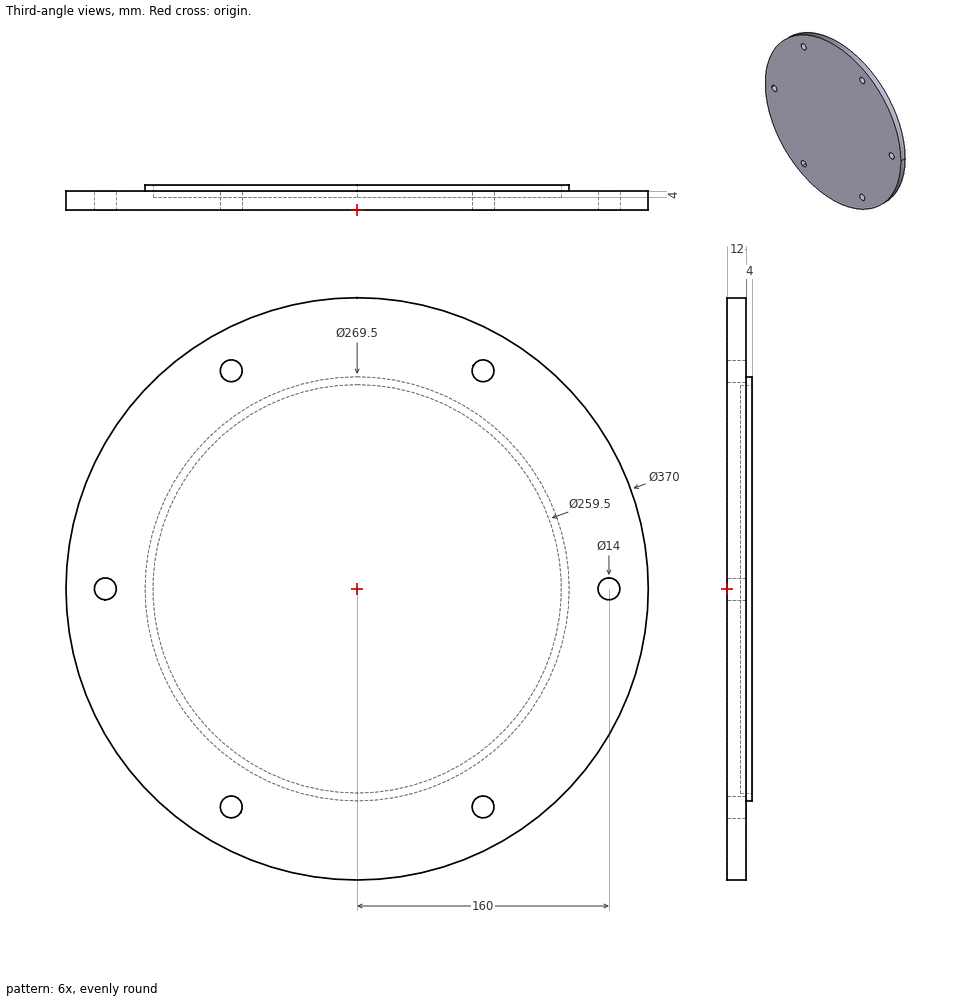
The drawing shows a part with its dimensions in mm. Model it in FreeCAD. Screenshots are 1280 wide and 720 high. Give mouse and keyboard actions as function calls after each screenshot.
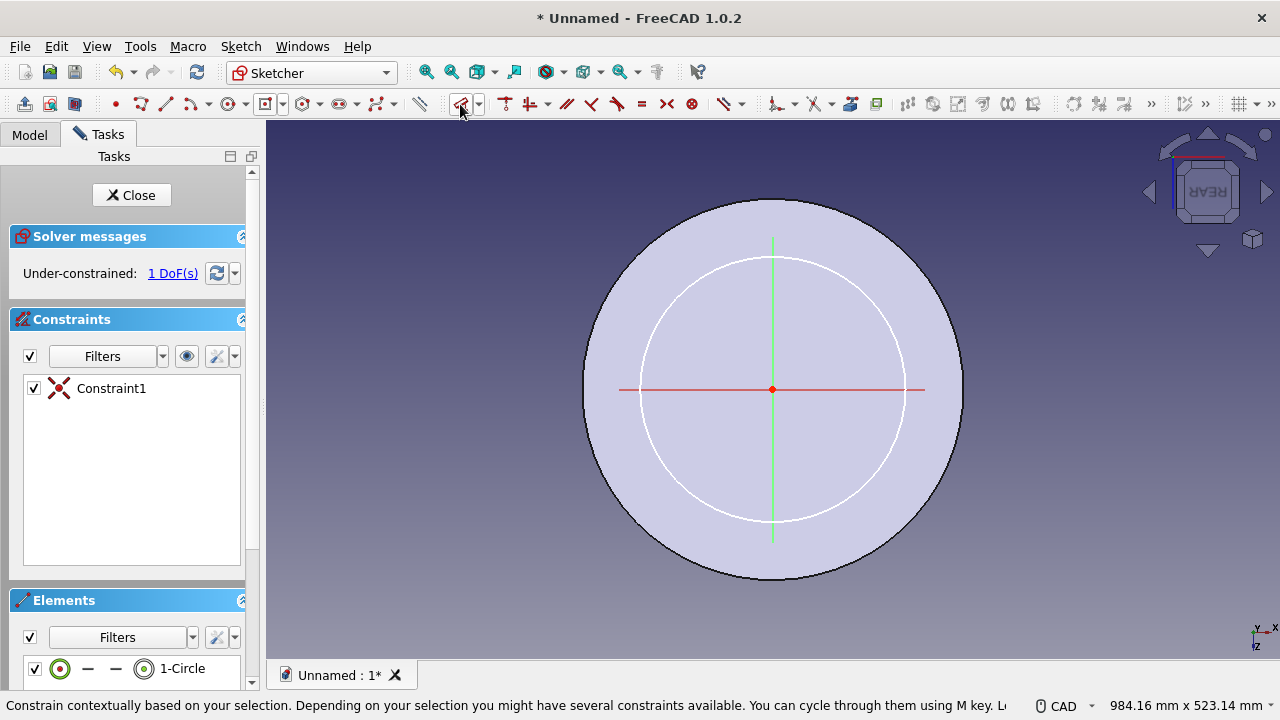
click(866, 295)
click(888, 272)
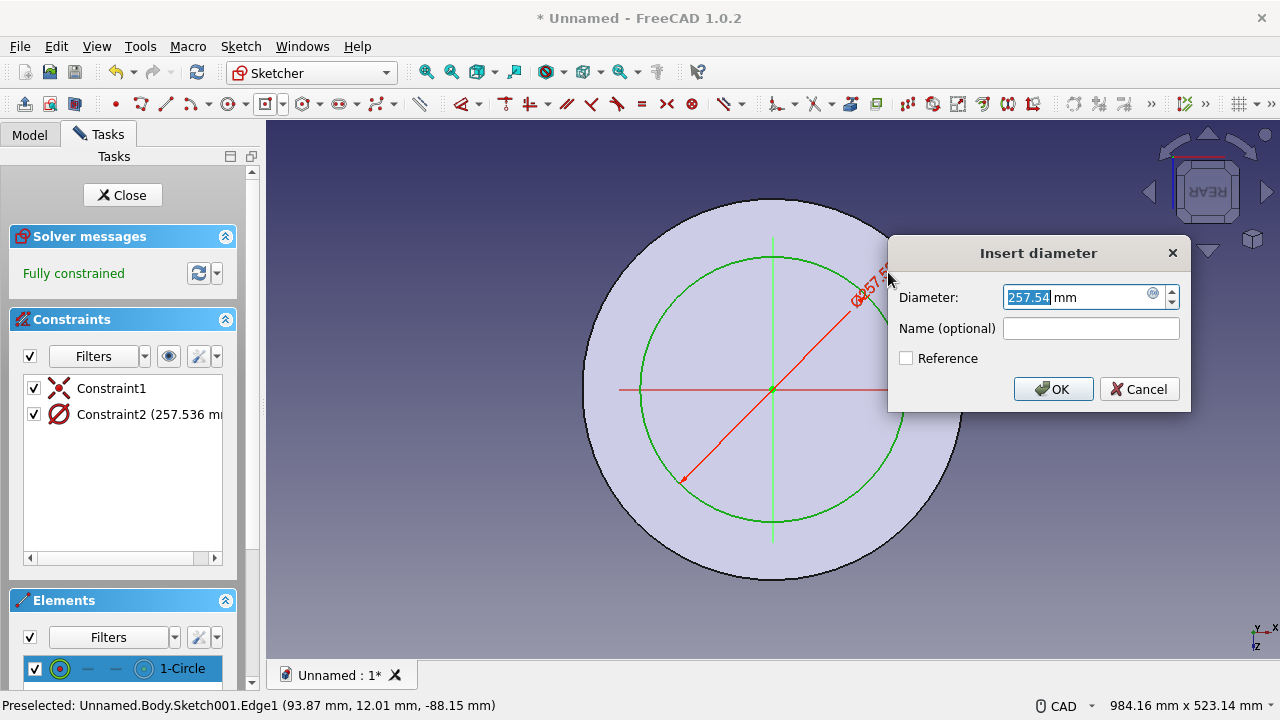
text(259.5)
key(Return)
key(Escape)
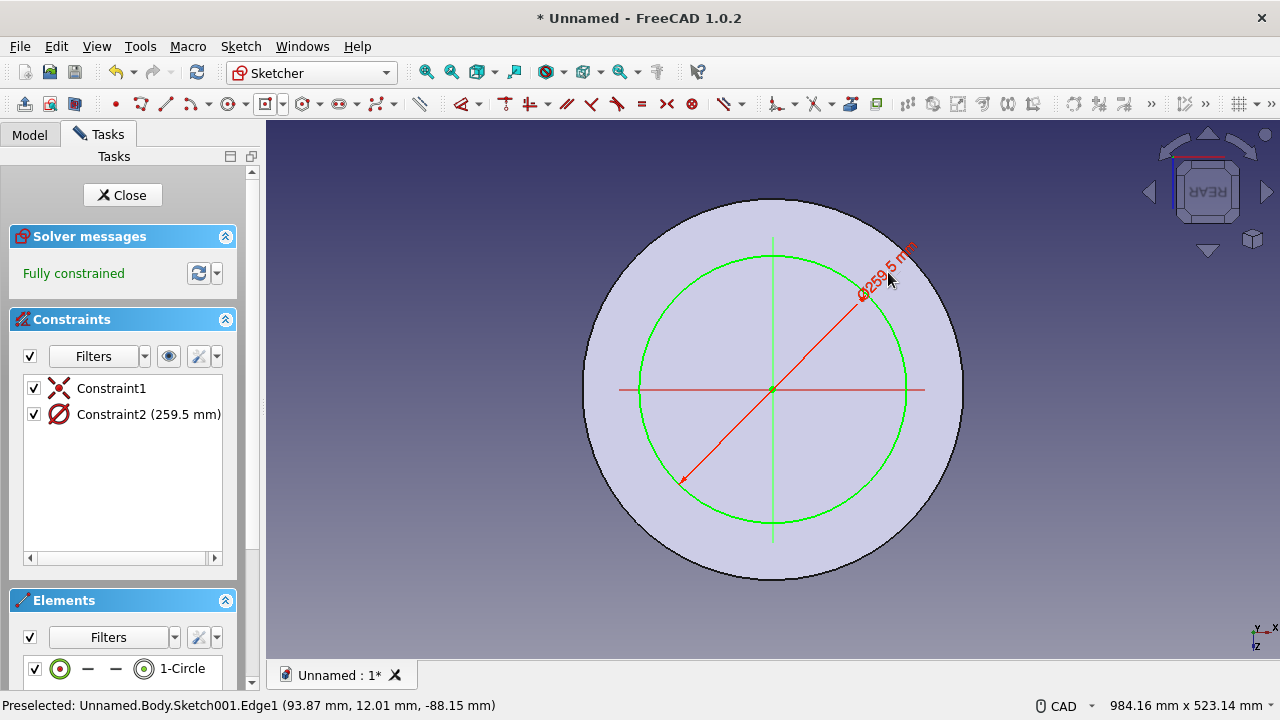
click(123, 195)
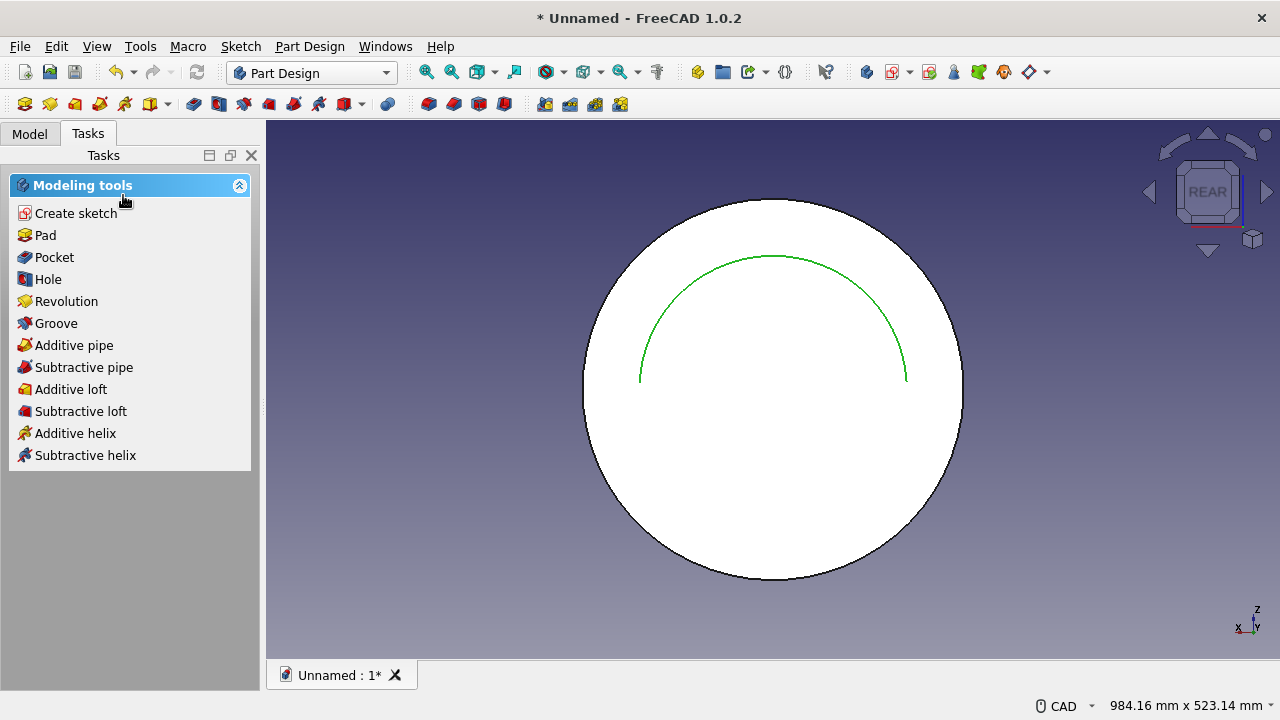
click(194, 104)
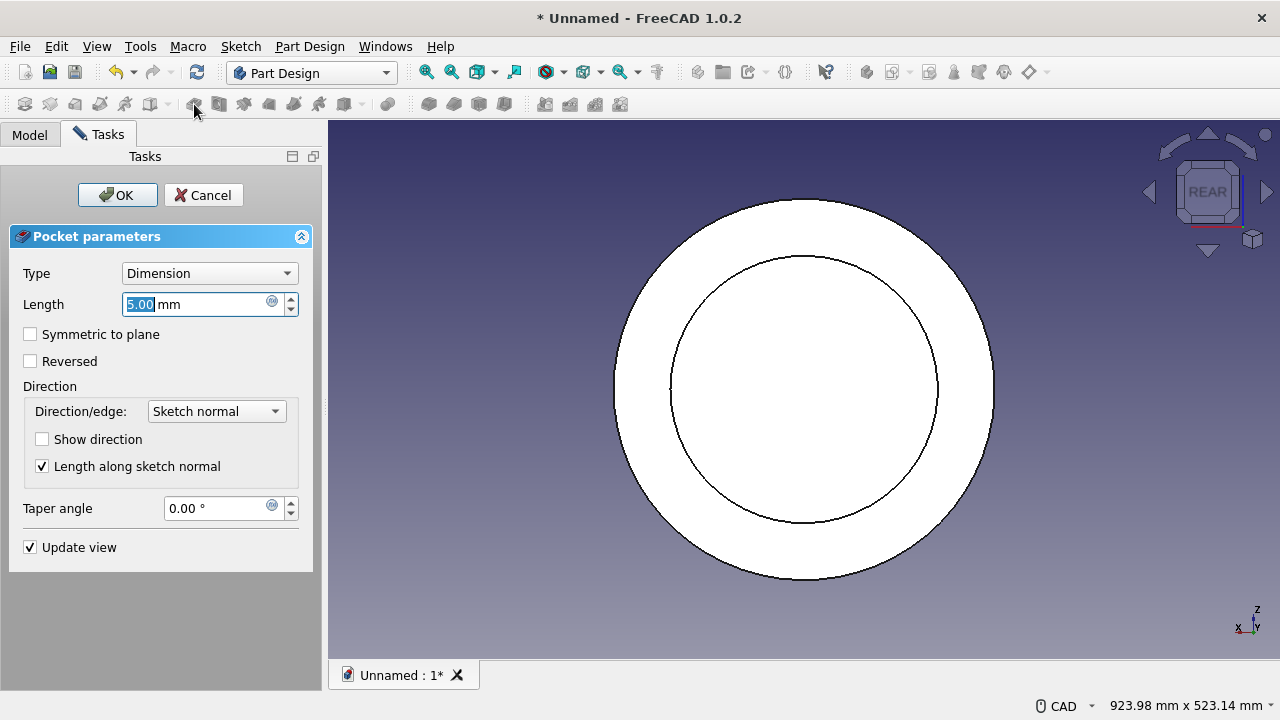
text(4)
key(Tab)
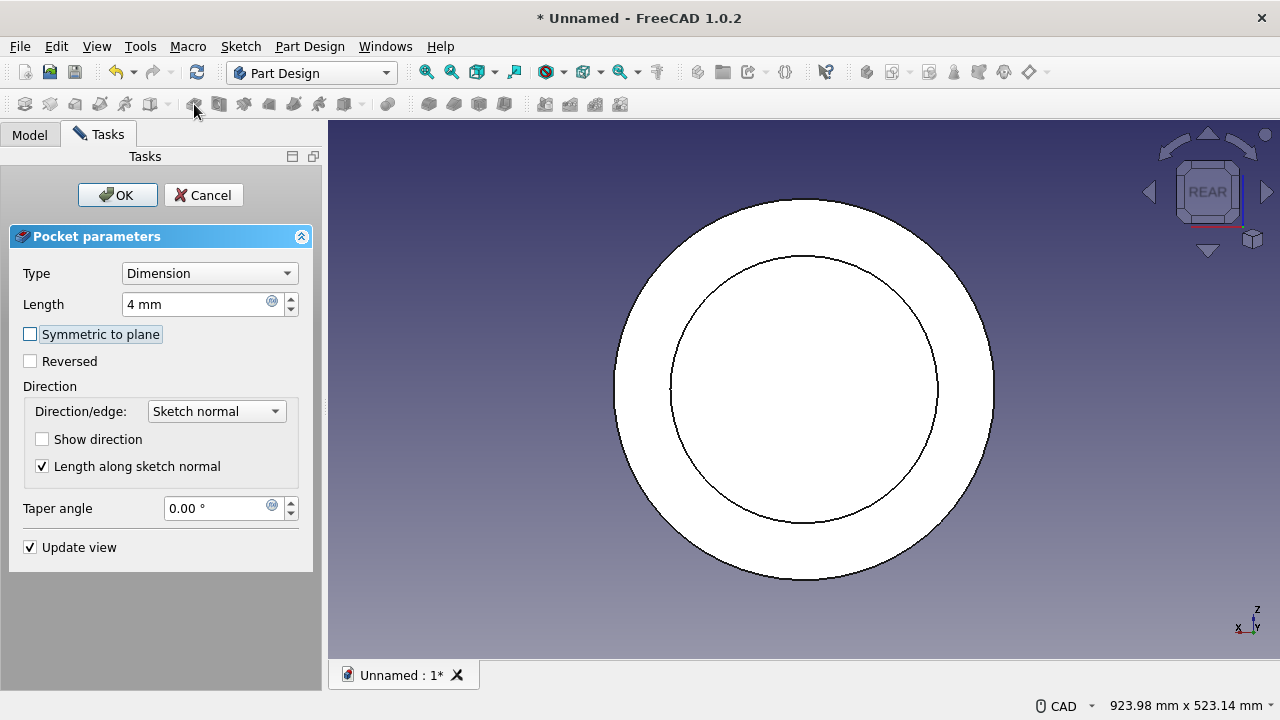
click(118, 195)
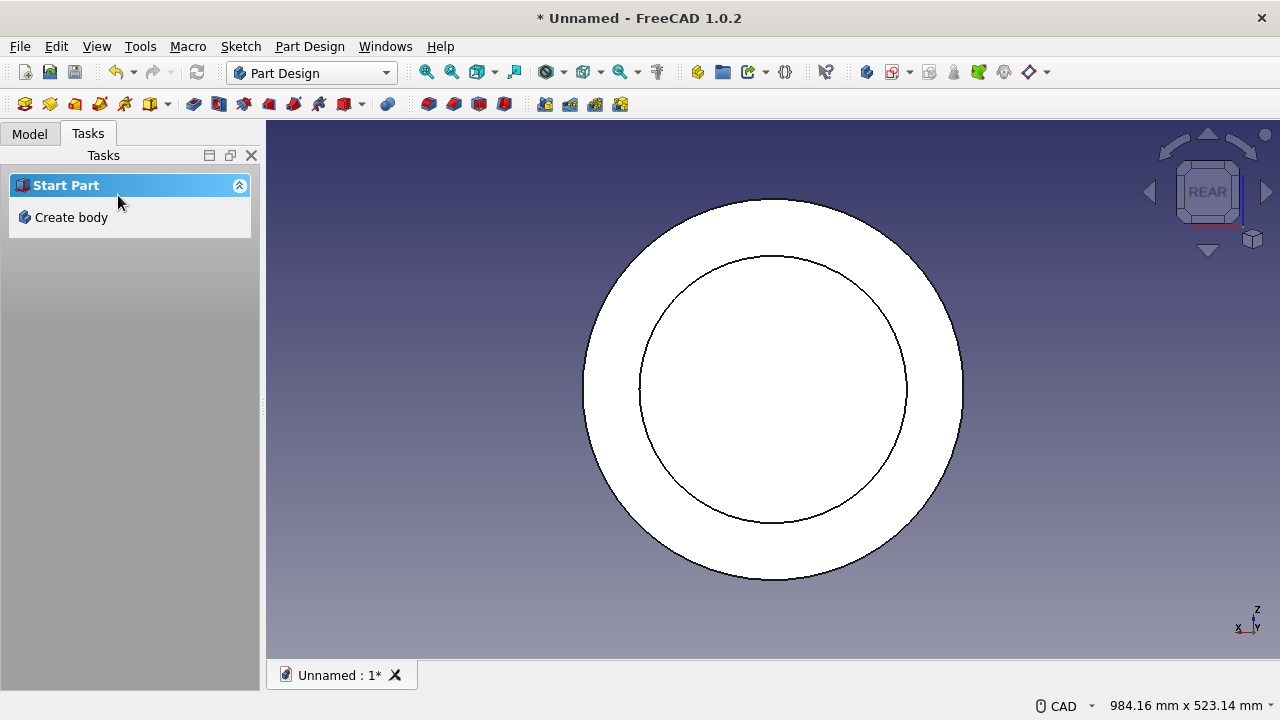
click(30, 134)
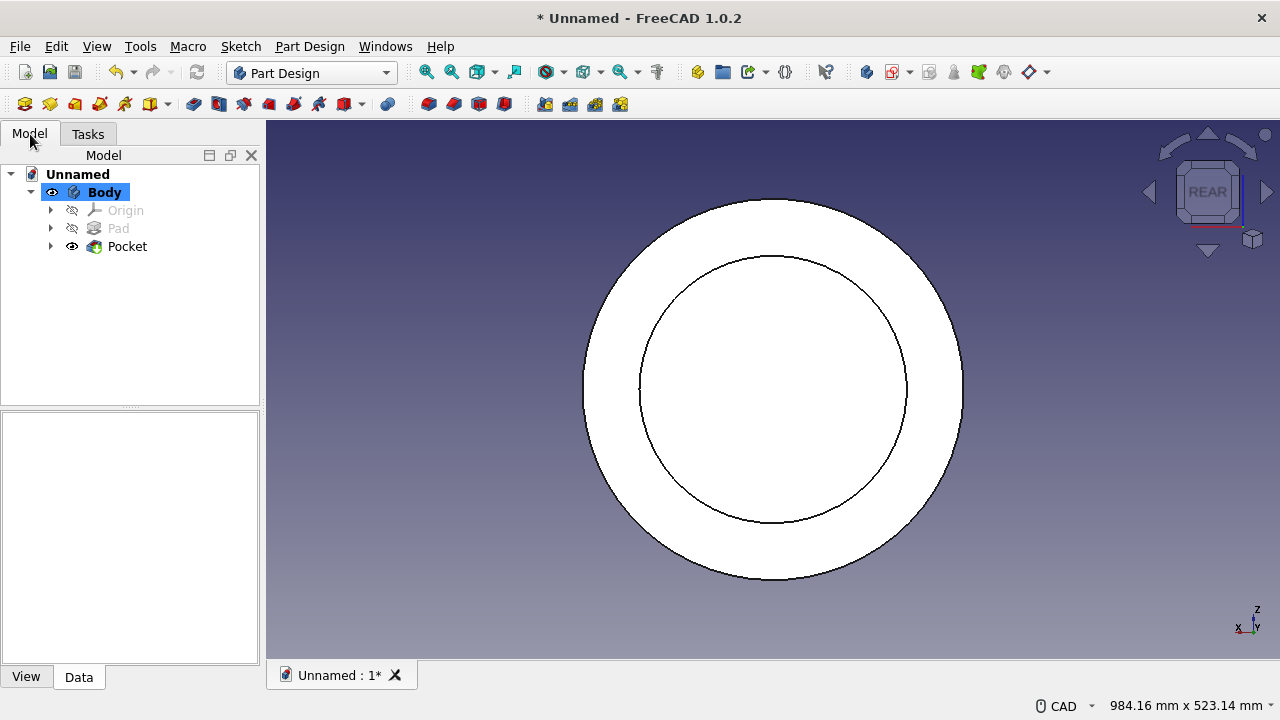
click(51, 210)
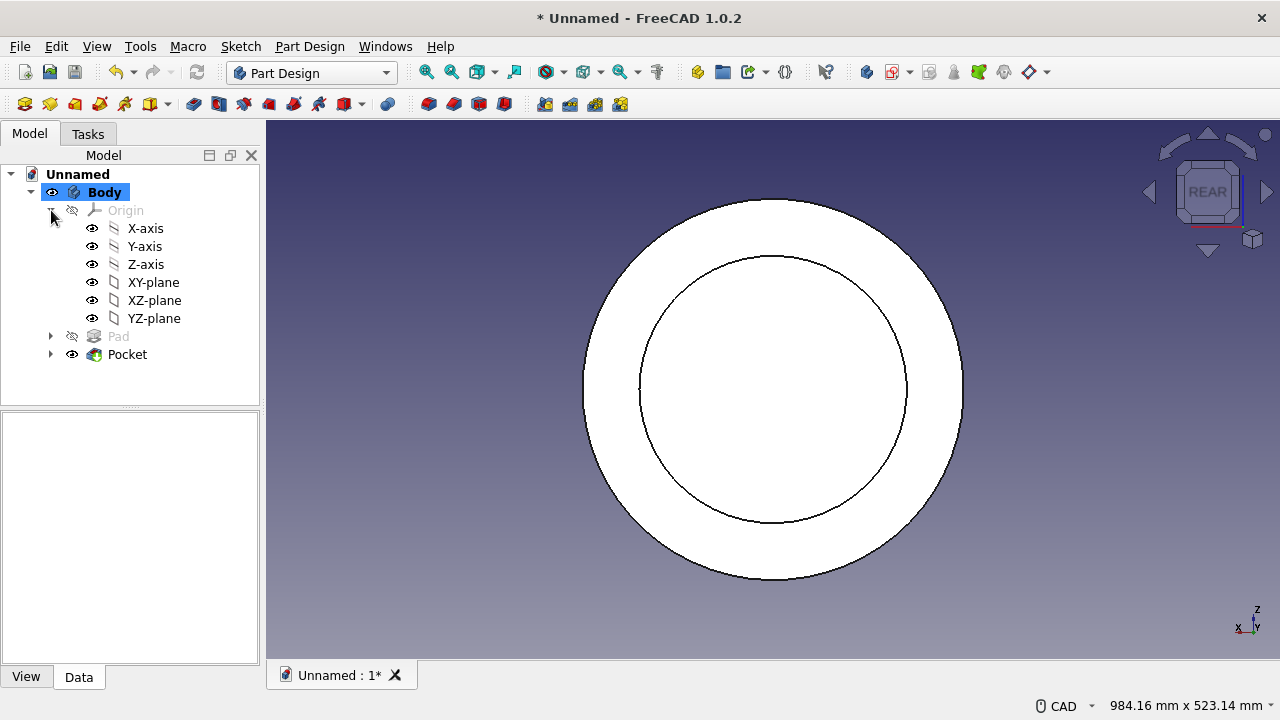
click(137, 300)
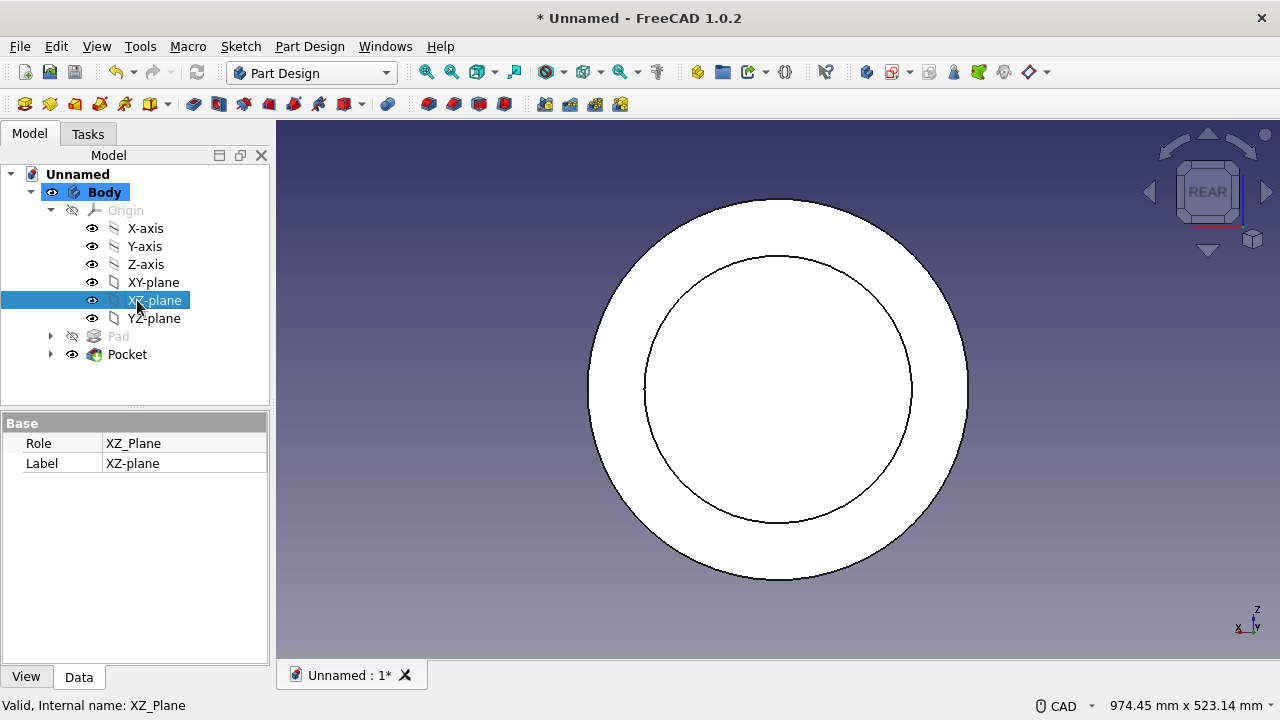
click(1028, 72)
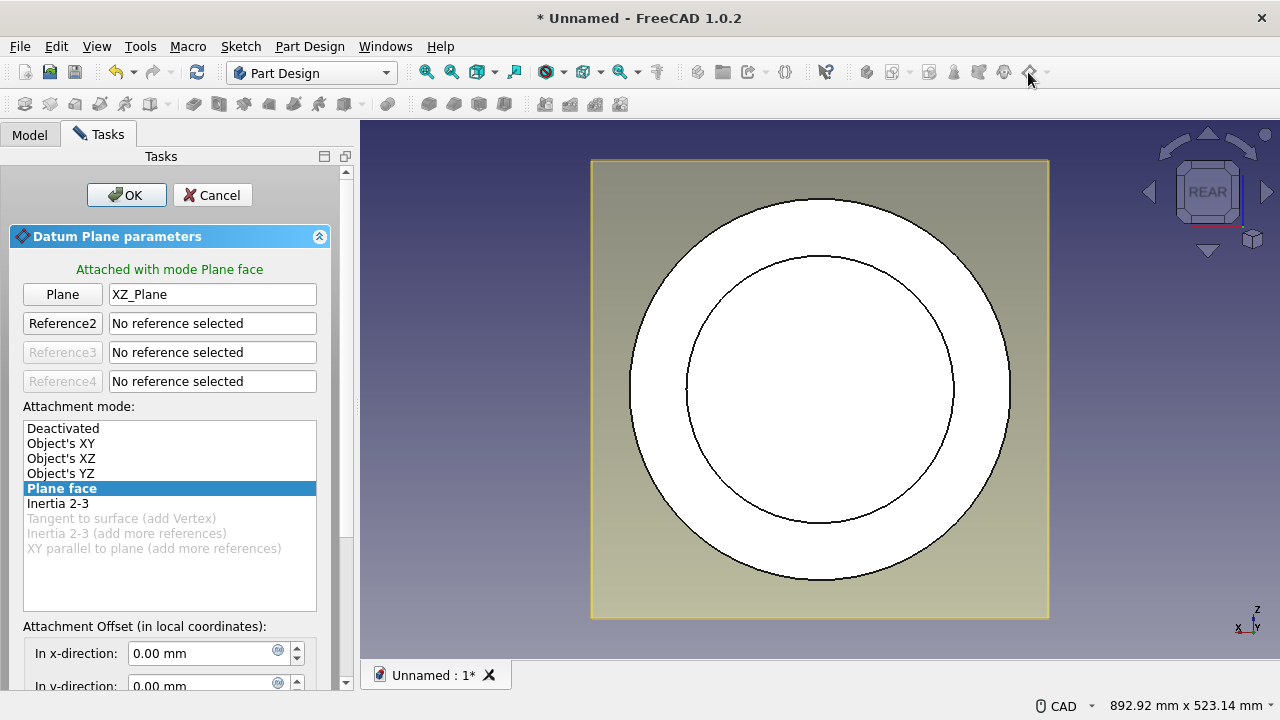
scroll(346, 428, down, 2)